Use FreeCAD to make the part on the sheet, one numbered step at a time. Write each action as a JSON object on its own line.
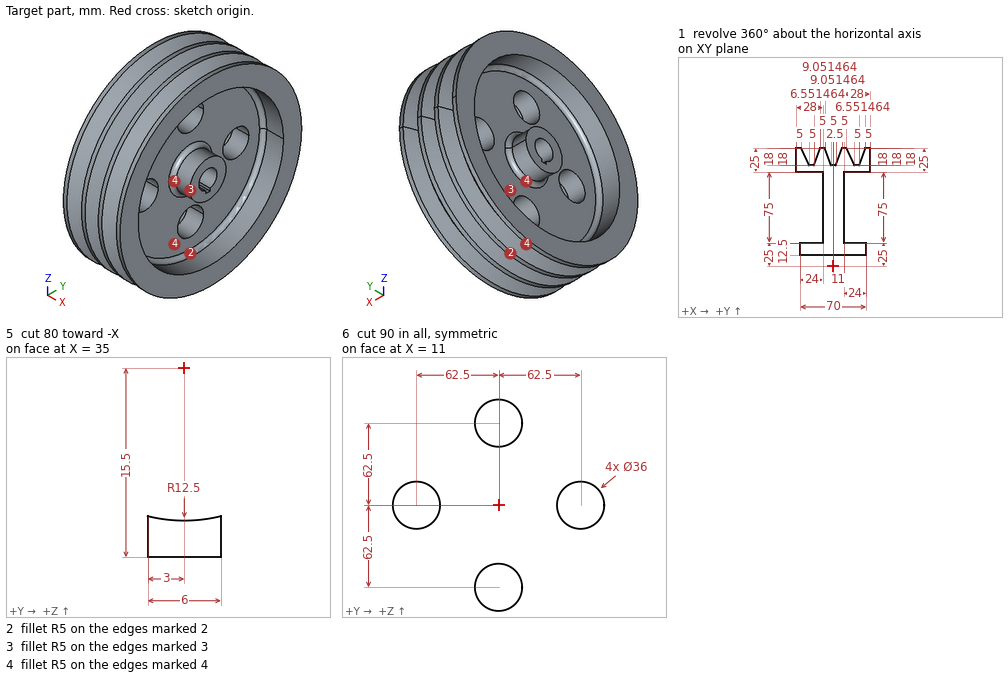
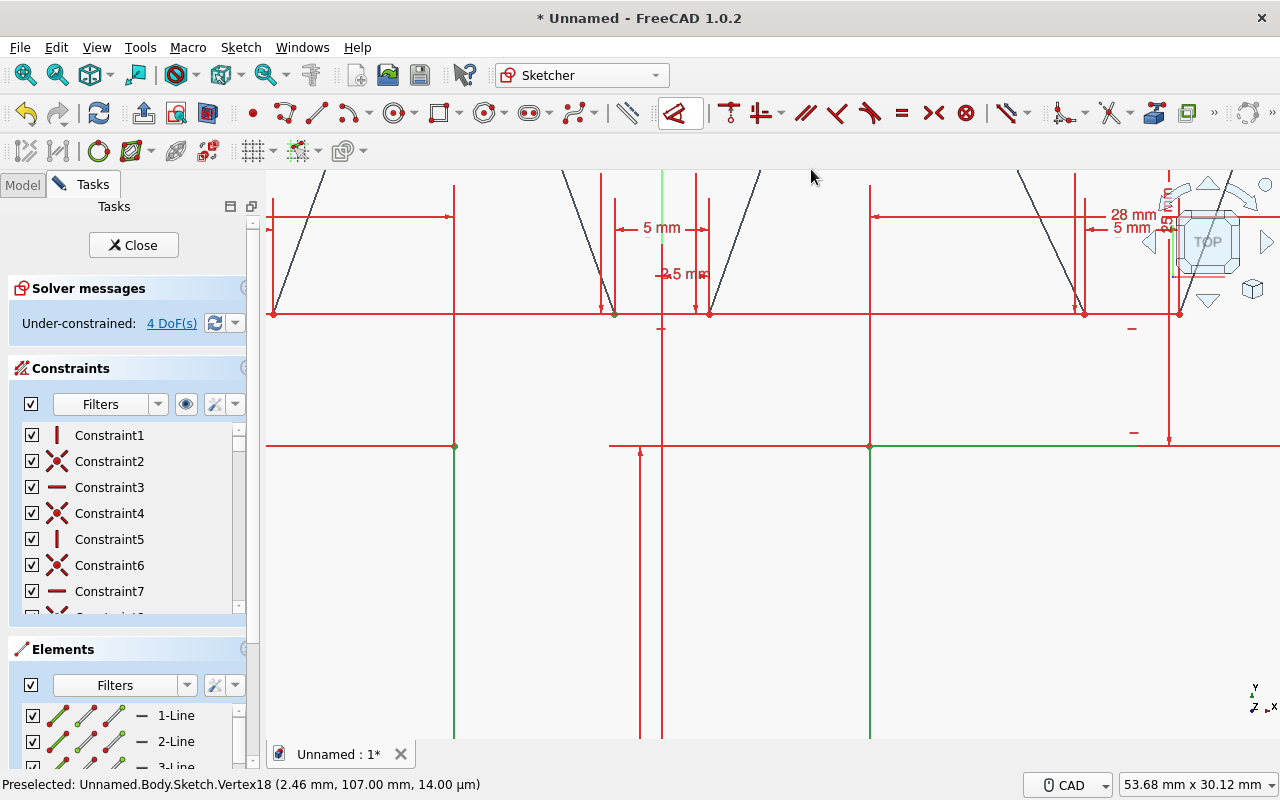
{"action": "scroll", "coordinate": [713, 316], "scroll_direction": "down", "scroll_amount": 9}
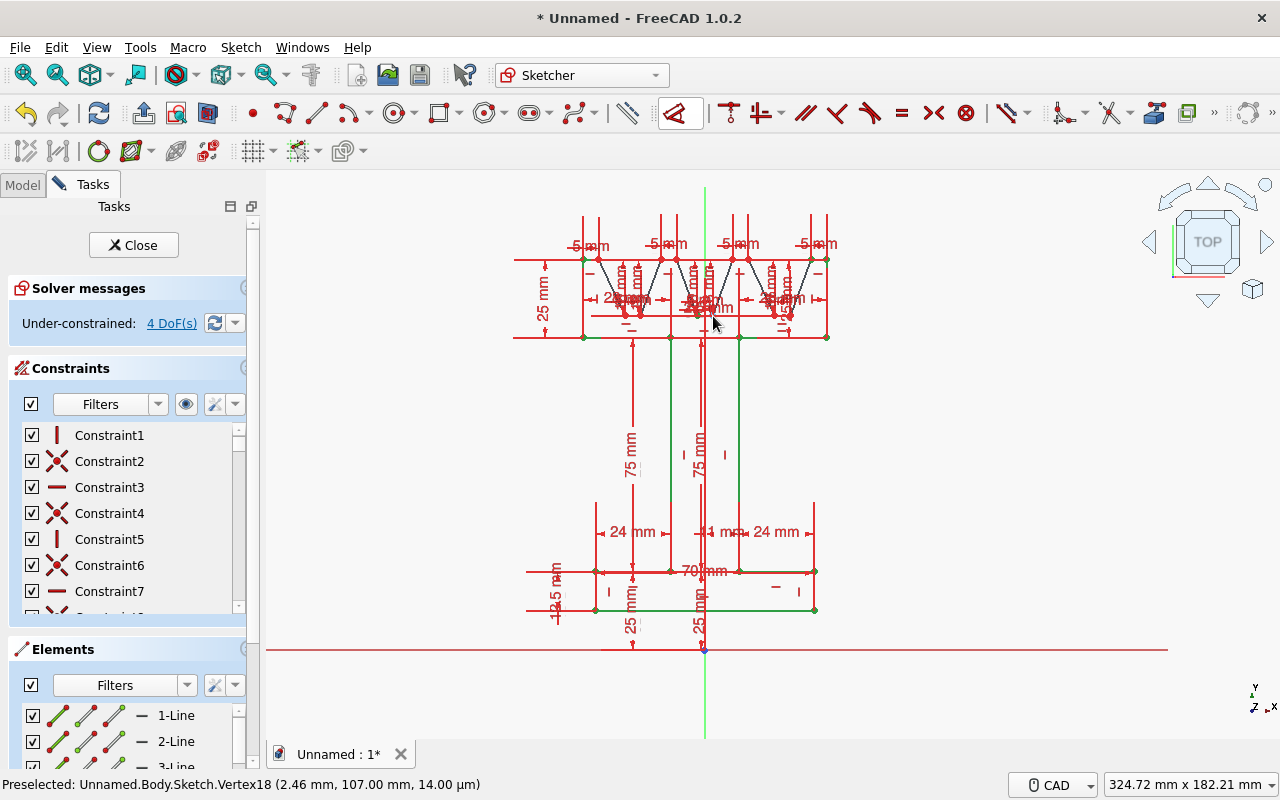
{"action": "scroll", "coordinate": [733, 260], "scroll_direction": "up", "scroll_amount": 2}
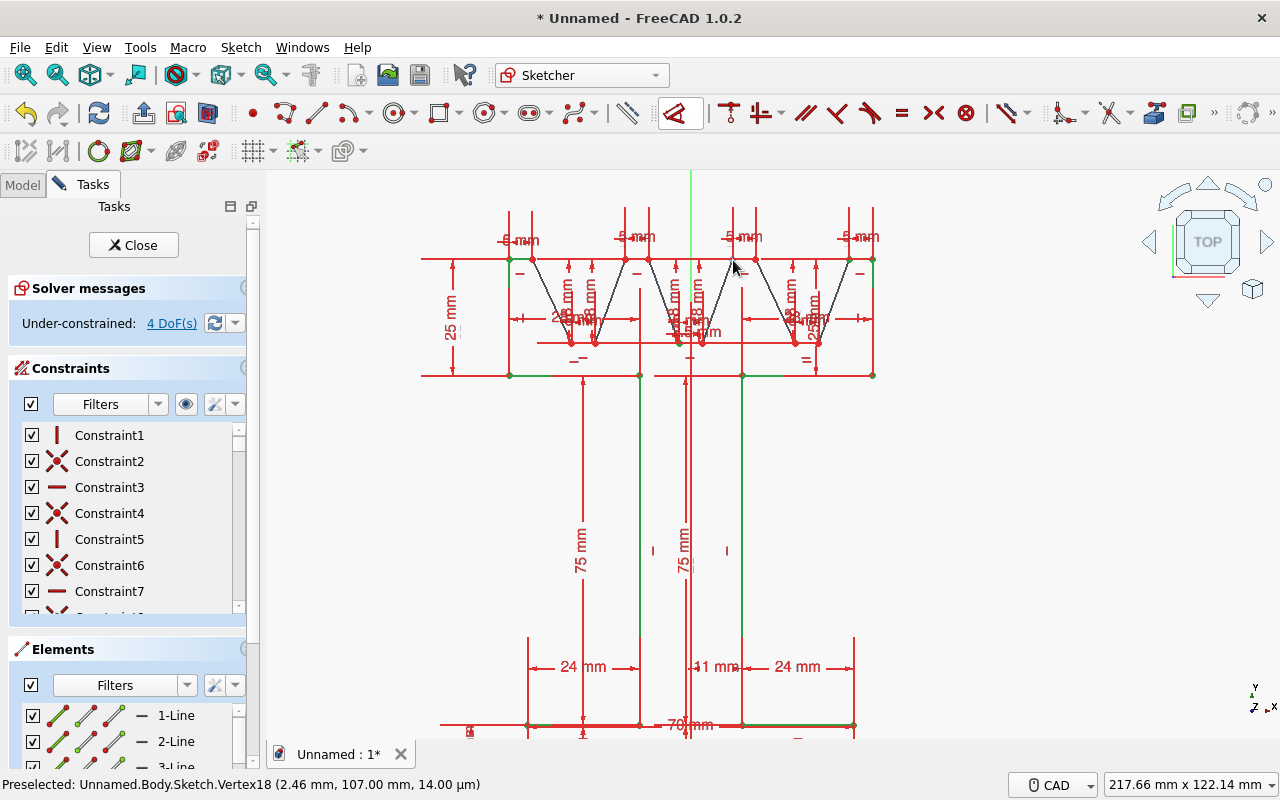
{"action": "left_click", "coordinate": [733, 259]}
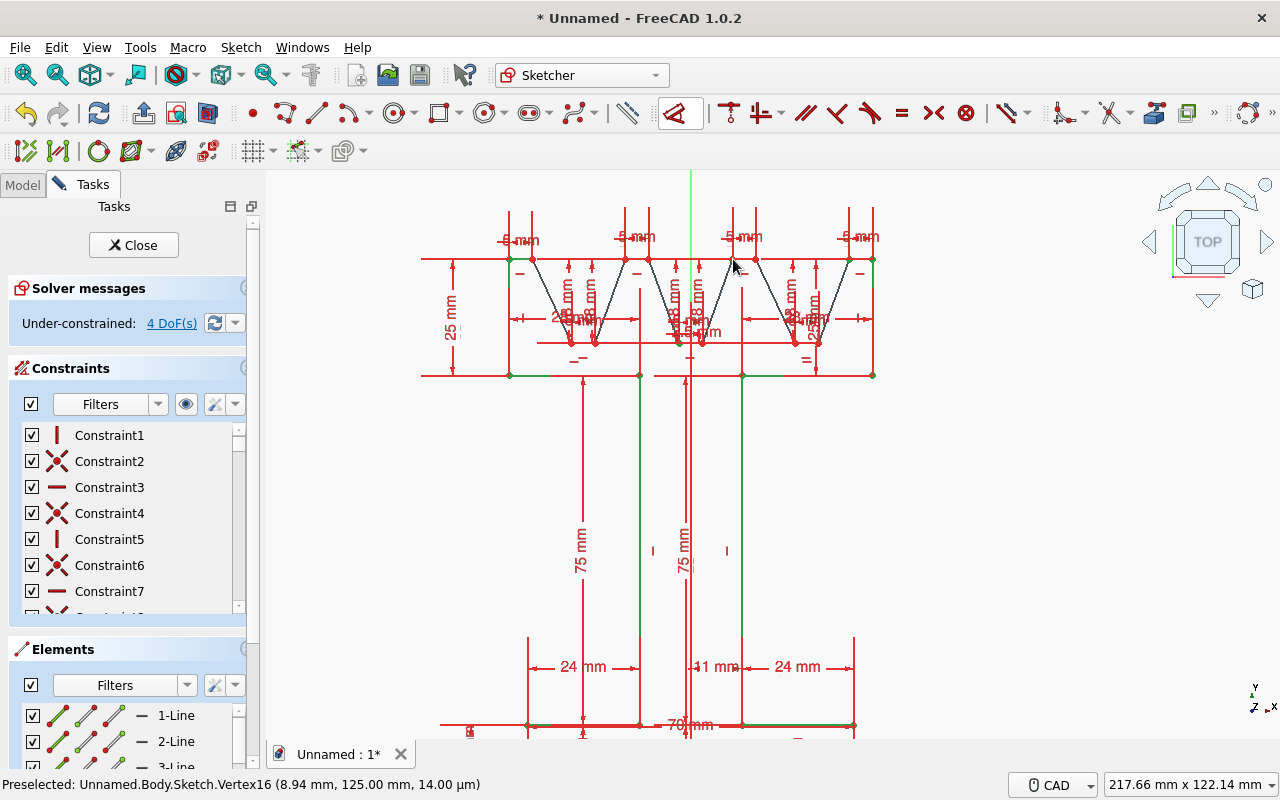
{"action": "left_click", "coordinate": [698, 114]}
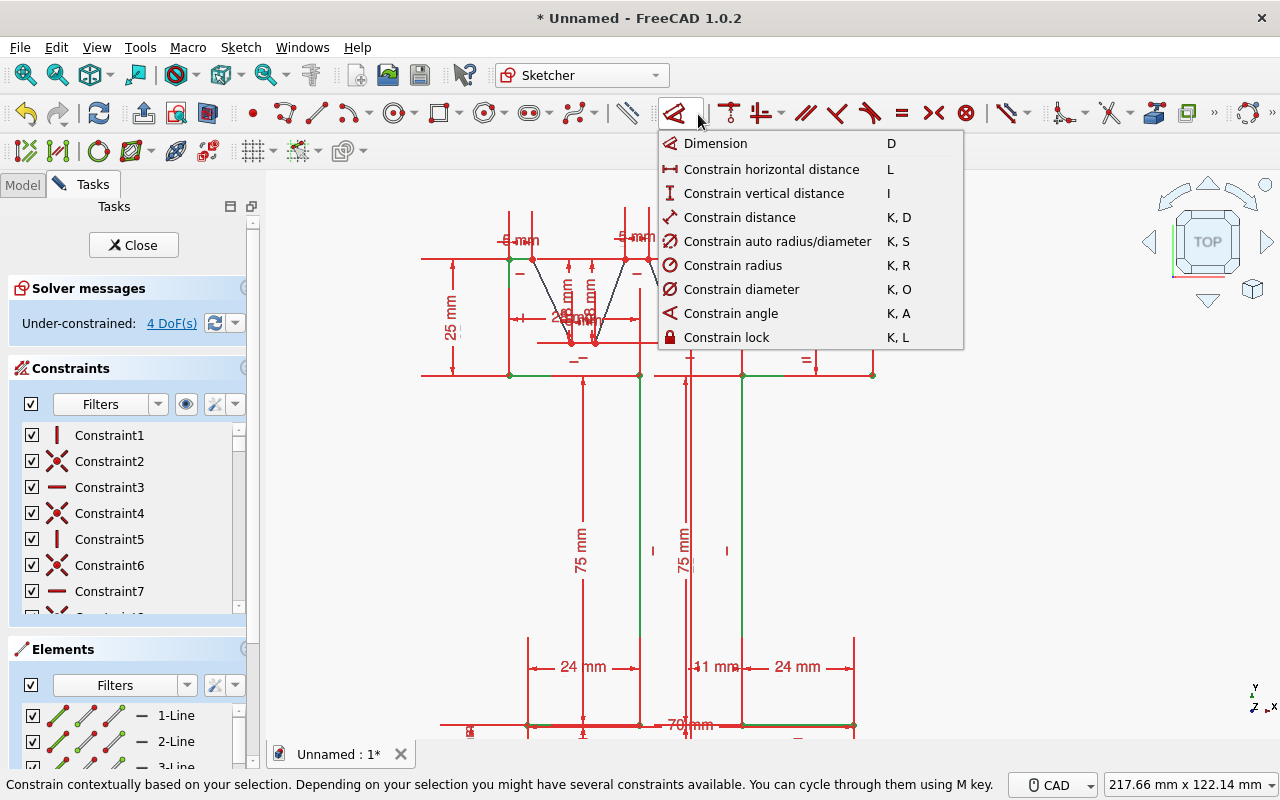
{"action": "left_click", "coordinate": [811, 169]}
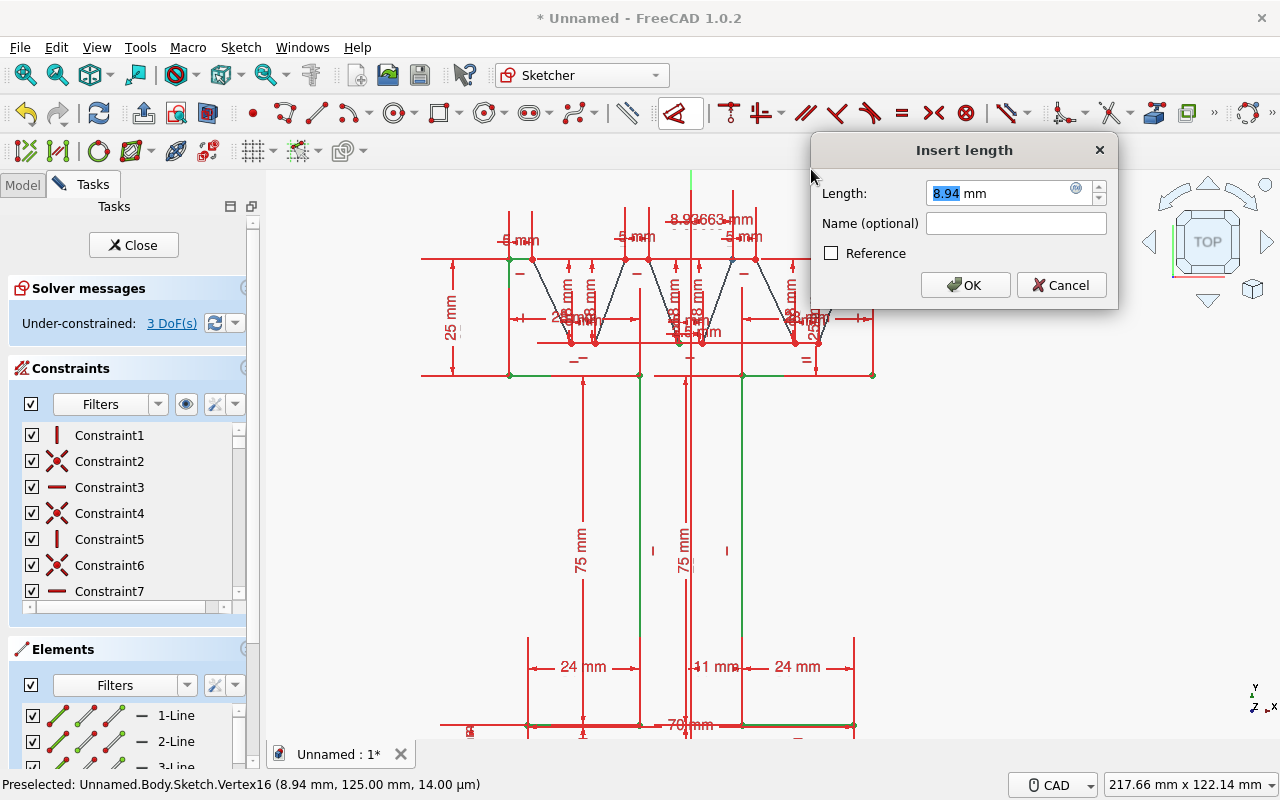
{"action": "type", "text": "9.051464"}
{"action": "key", "text": "Return"}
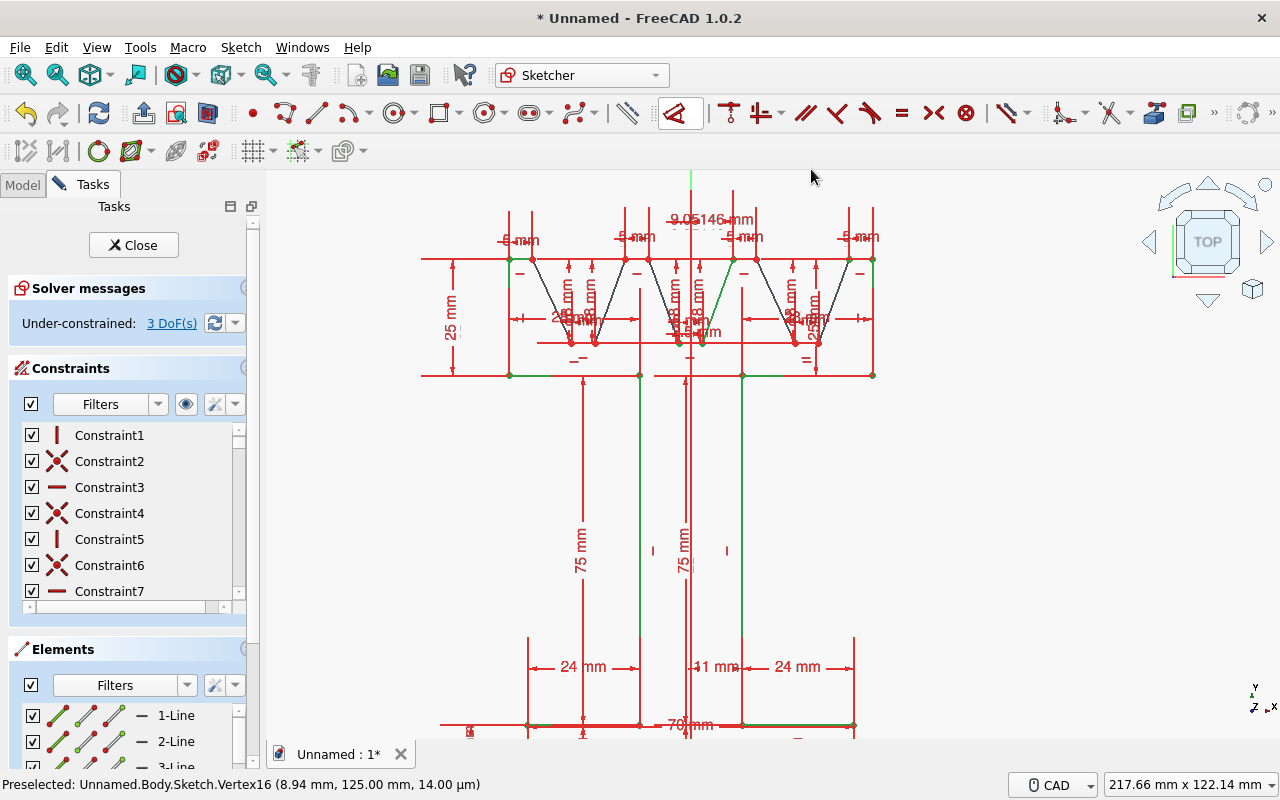
{"action": "left_click", "coordinate": [649, 259]}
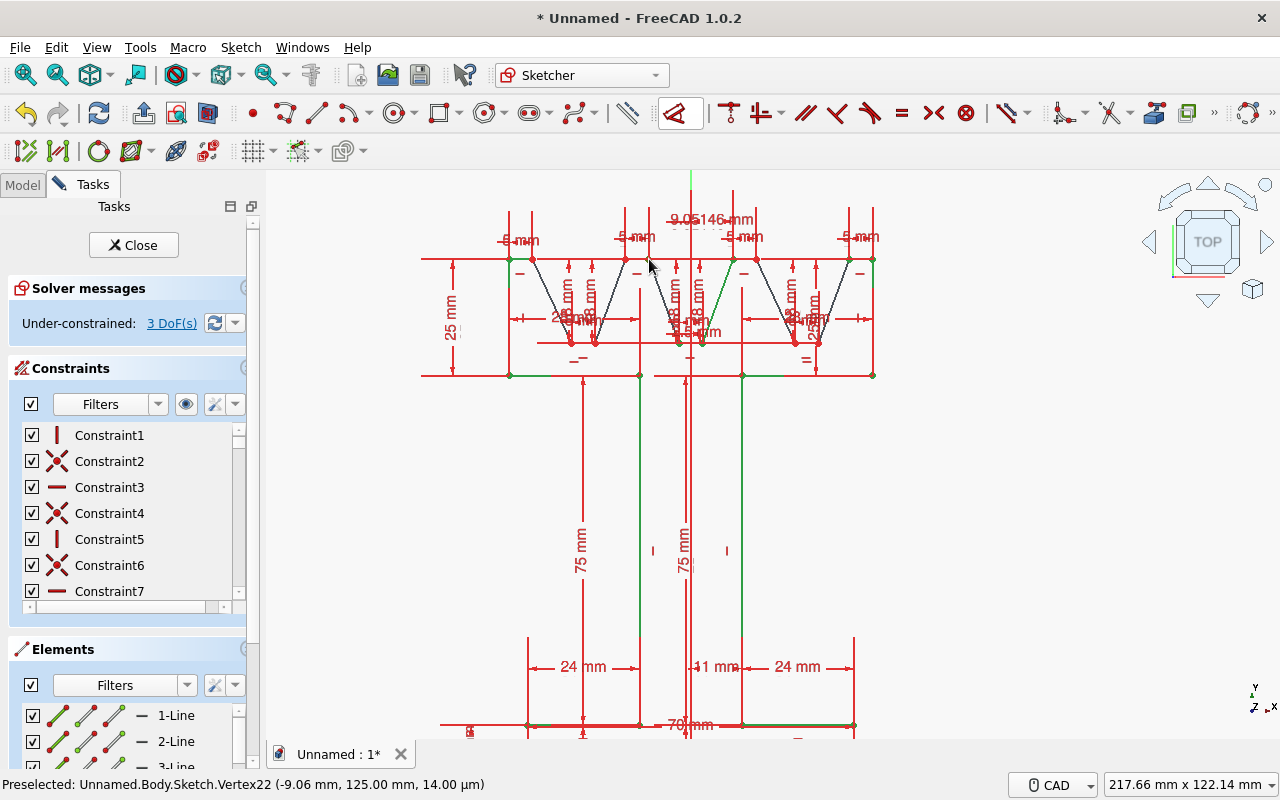
{"action": "key", "text": "l"}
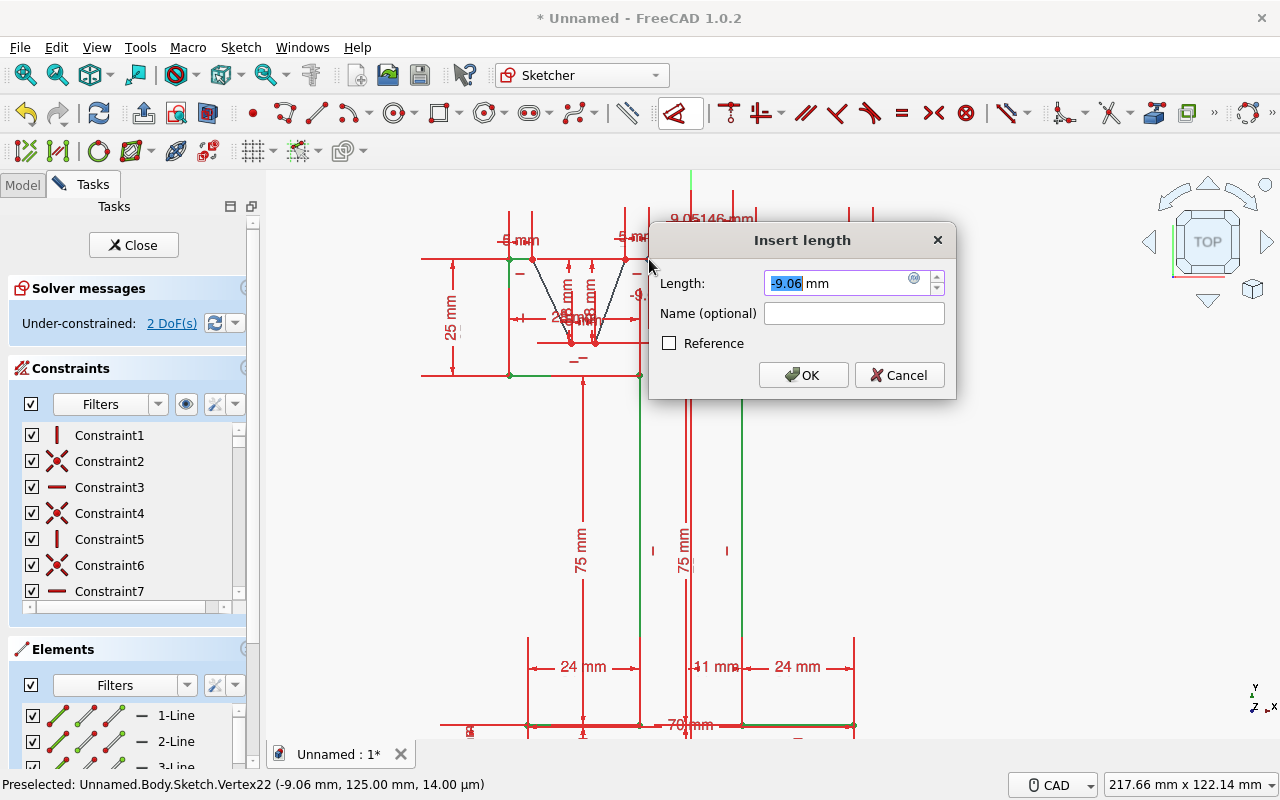
{"action": "type", "text": "-9.051464"}
{"action": "key", "text": "Return"}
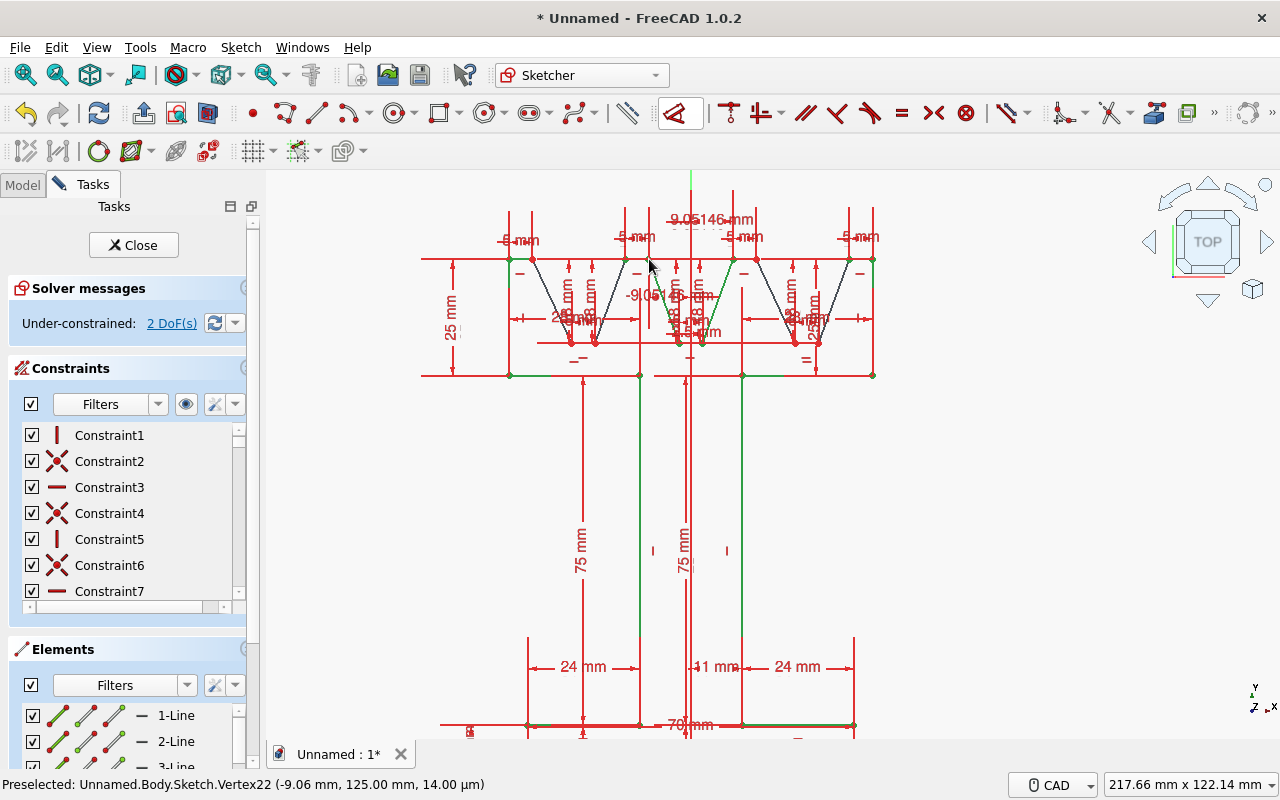
{"action": "scroll", "coordinate": [840, 285], "scroll_direction": "up", "scroll_amount": 2}